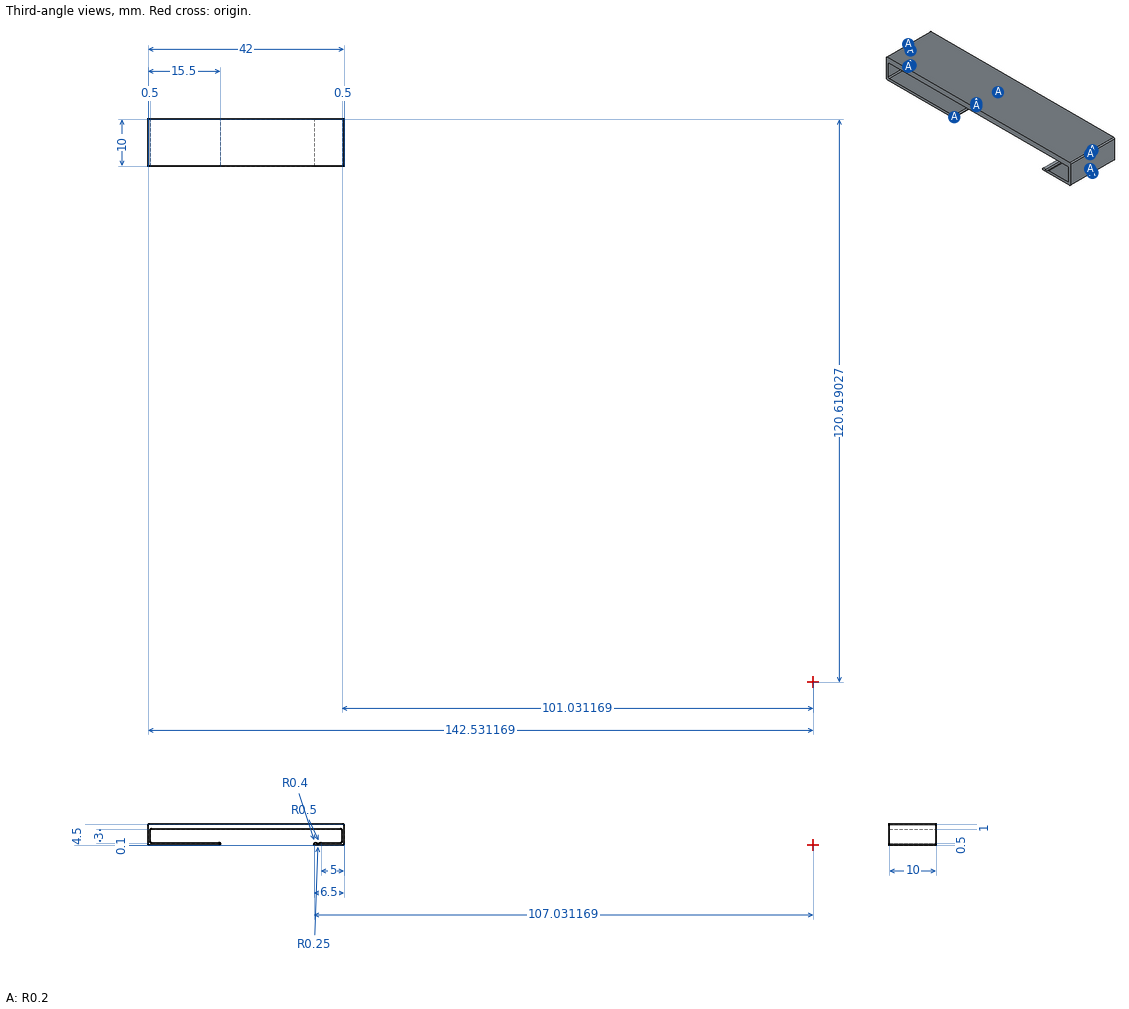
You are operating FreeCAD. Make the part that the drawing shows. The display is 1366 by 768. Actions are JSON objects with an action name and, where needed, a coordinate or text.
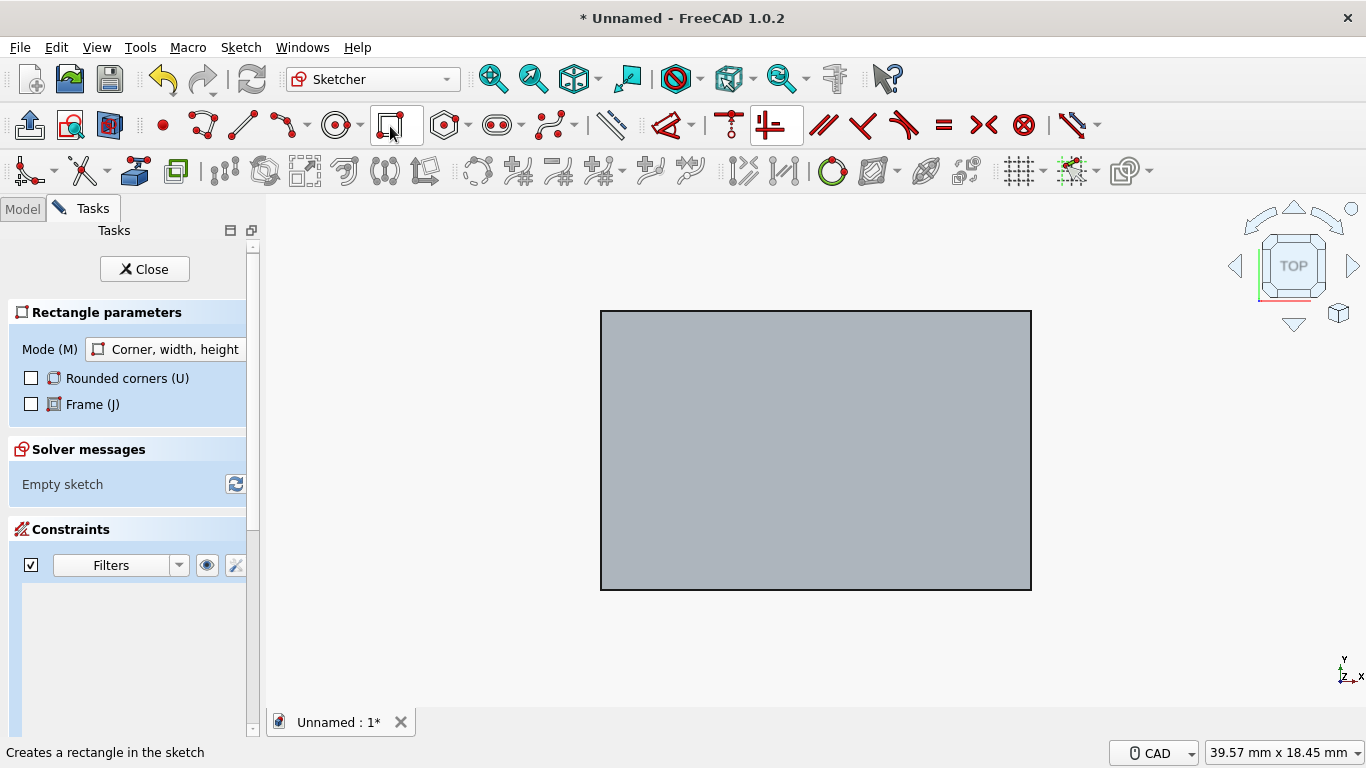
{"action": "left_click", "coordinate": [601, 311]}
{"action": "left_click", "coordinate": [614, 590]}
{"action": "key", "text": "Escape"}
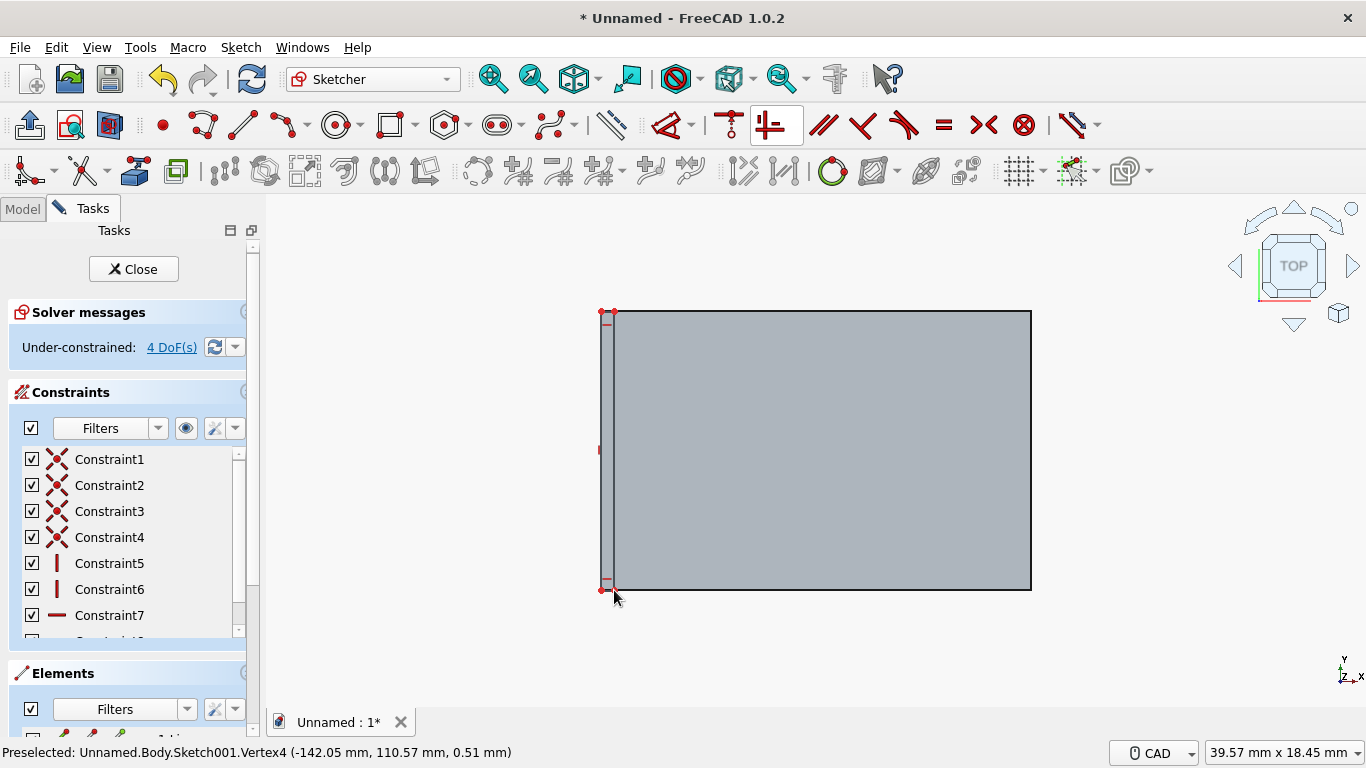
{"action": "left_click", "coordinate": [666, 126]}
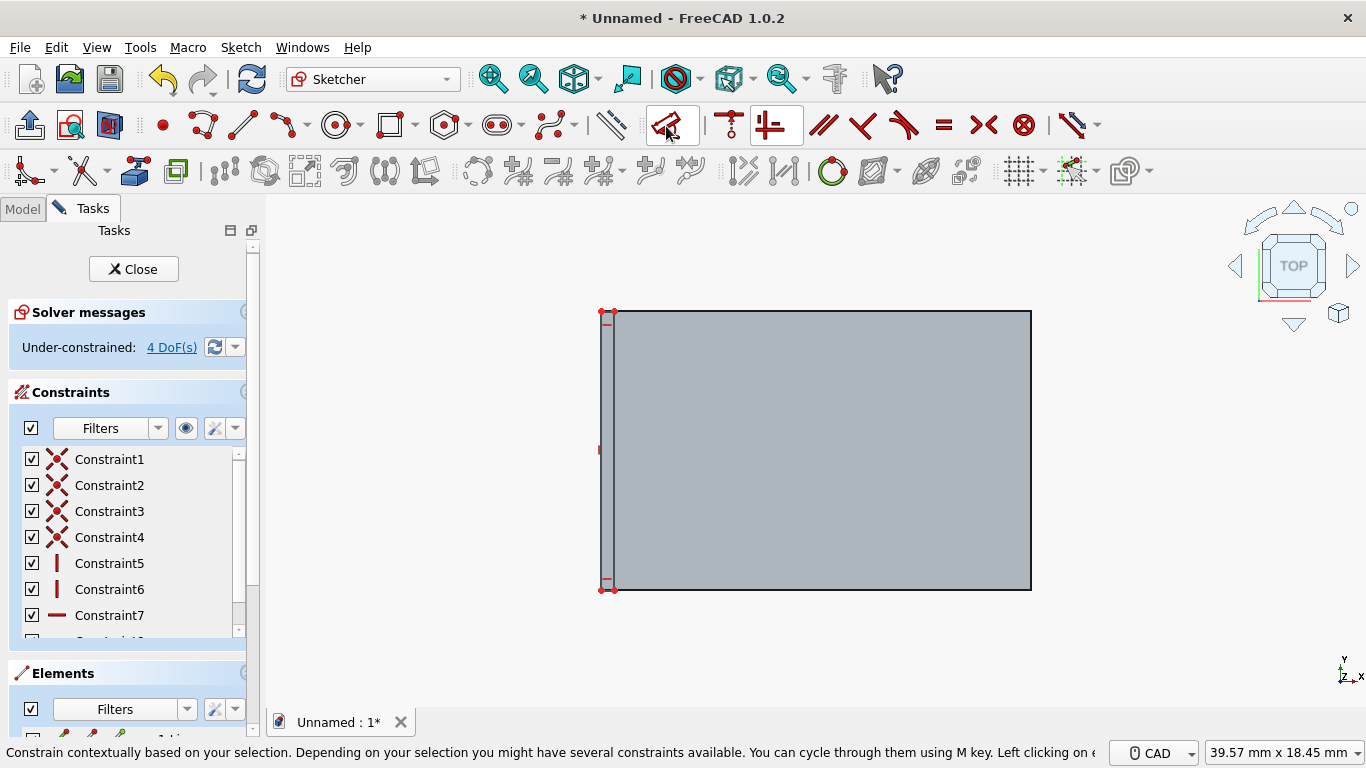
{"action": "left_click", "coordinate": [601, 396]}
{"action": "left_click", "coordinate": [567, 451]}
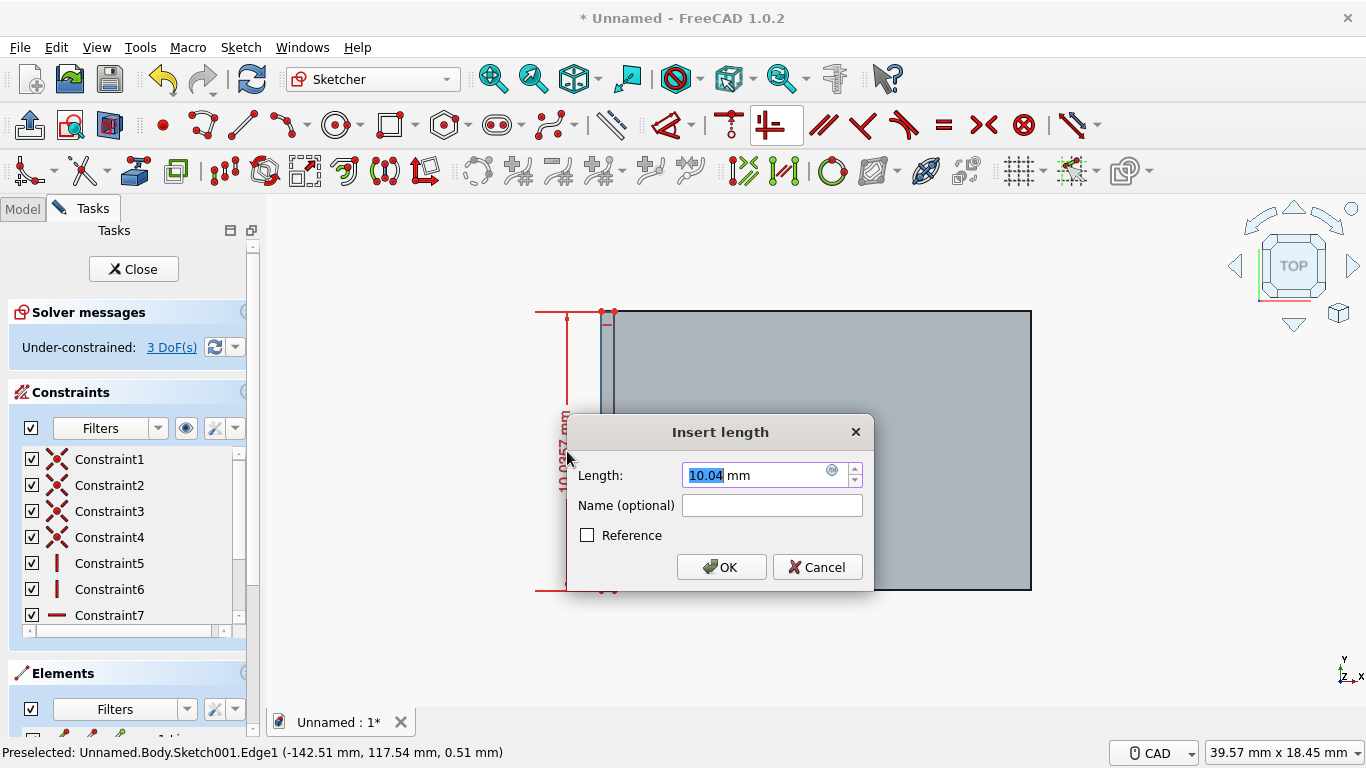
{"action": "type", "text": "10"}
{"action": "key", "text": "Return"}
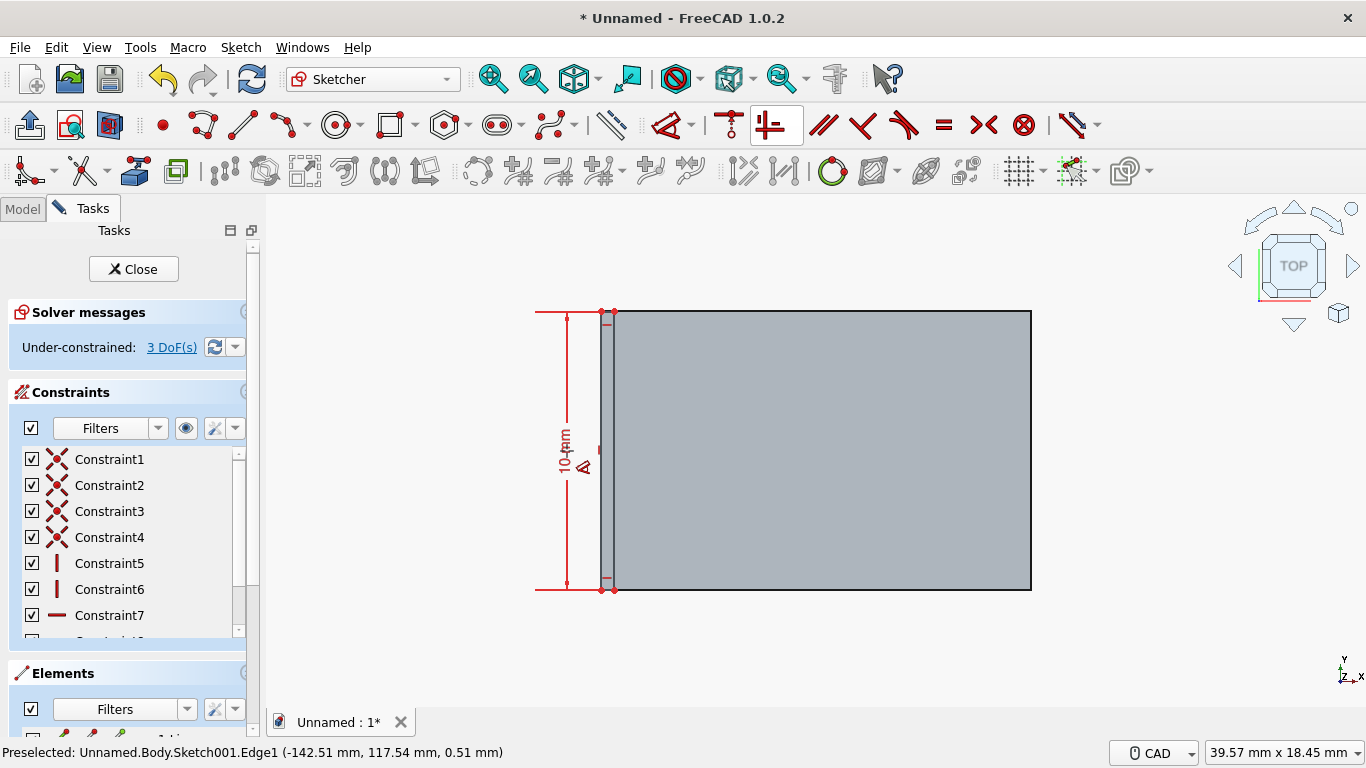
{"action": "scroll", "coordinate": [607, 590], "scroll_direction": "up", "scroll_amount": 6}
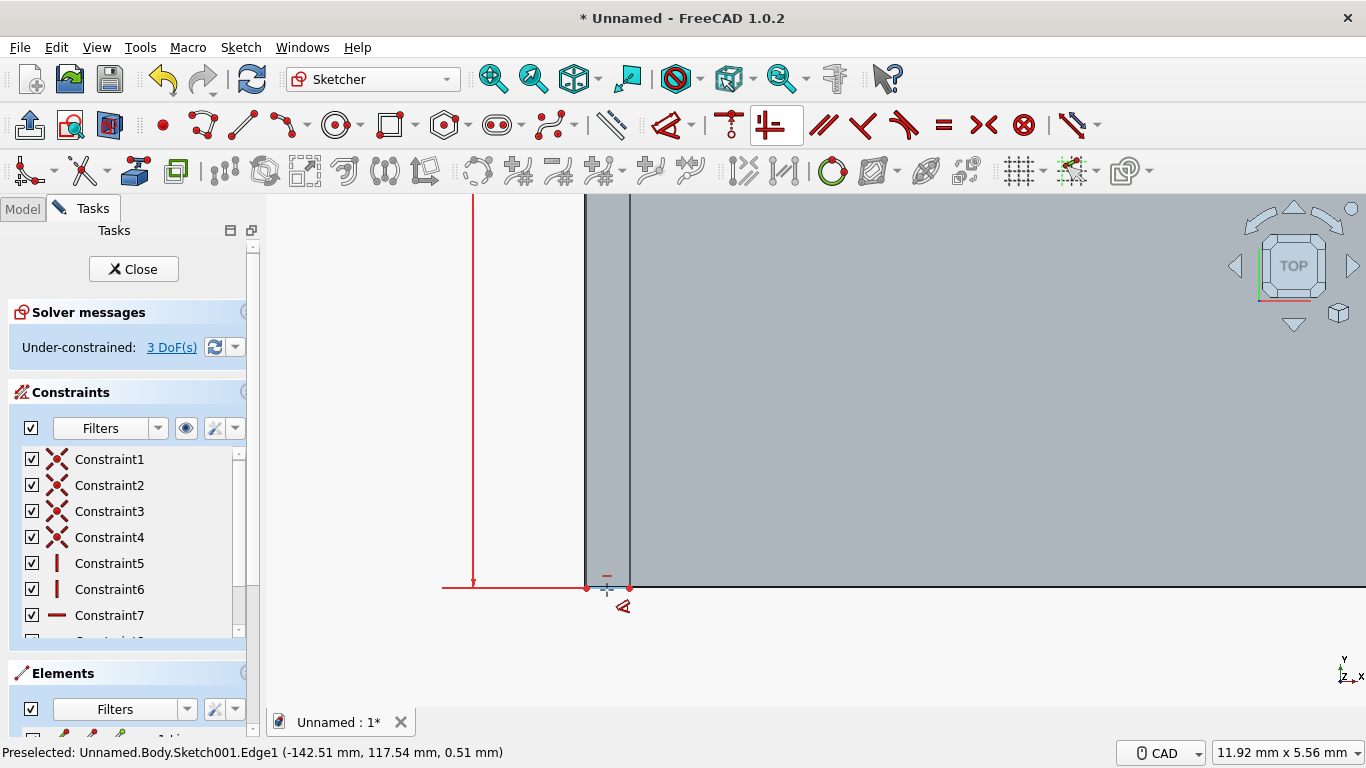
{"action": "left_click", "coordinate": [608, 588]}
{"action": "left_click", "coordinate": [608, 622]}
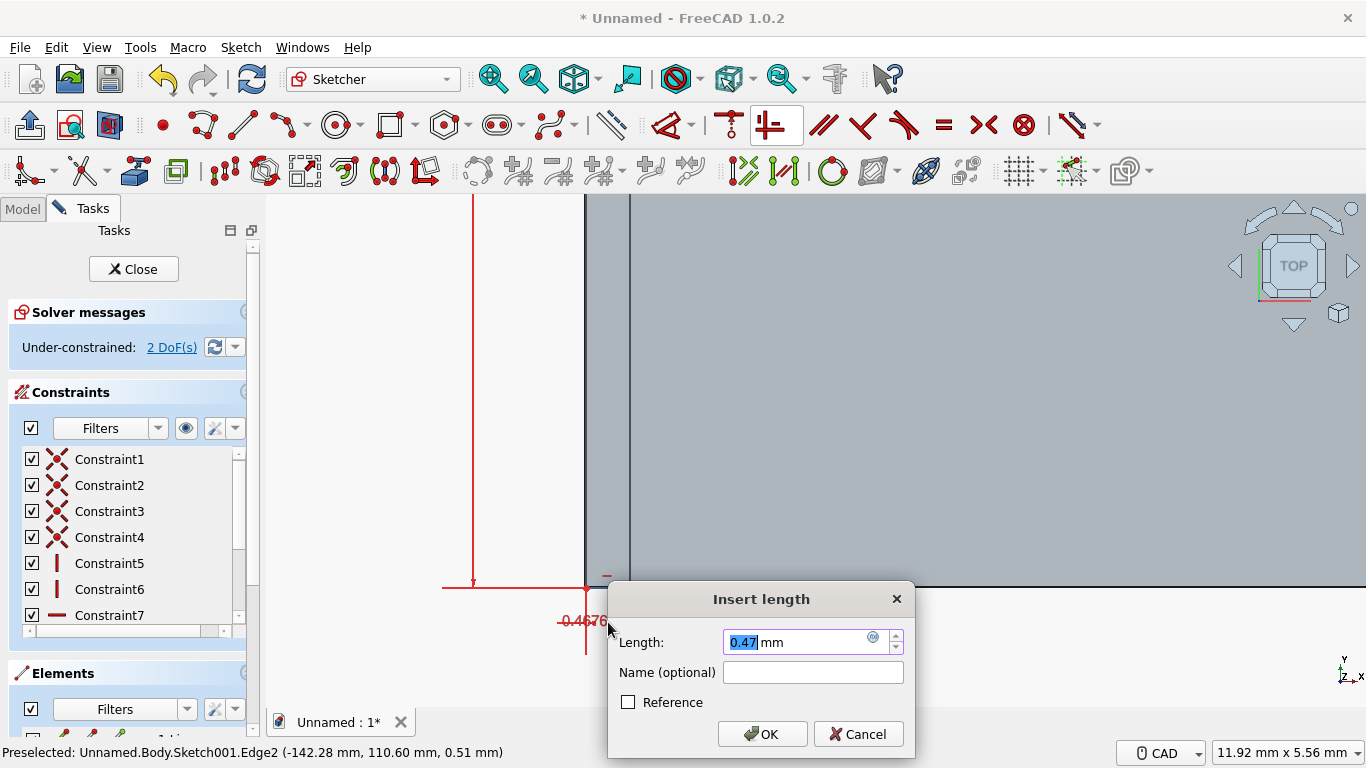
{"action": "type", "text": "0.5"}
{"action": "key", "text": "Return"}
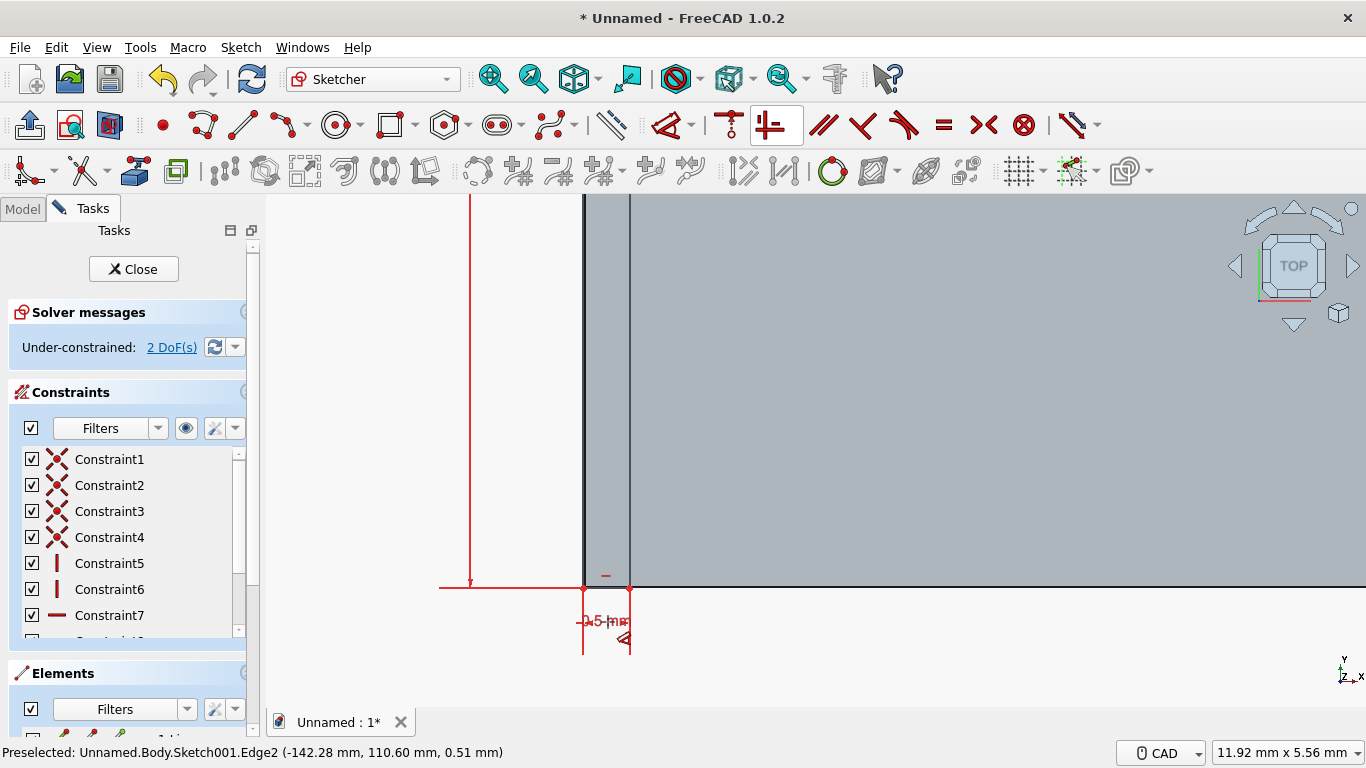
{"action": "scroll", "coordinate": [829, 640], "scroll_direction": "down", "scroll_amount": 5}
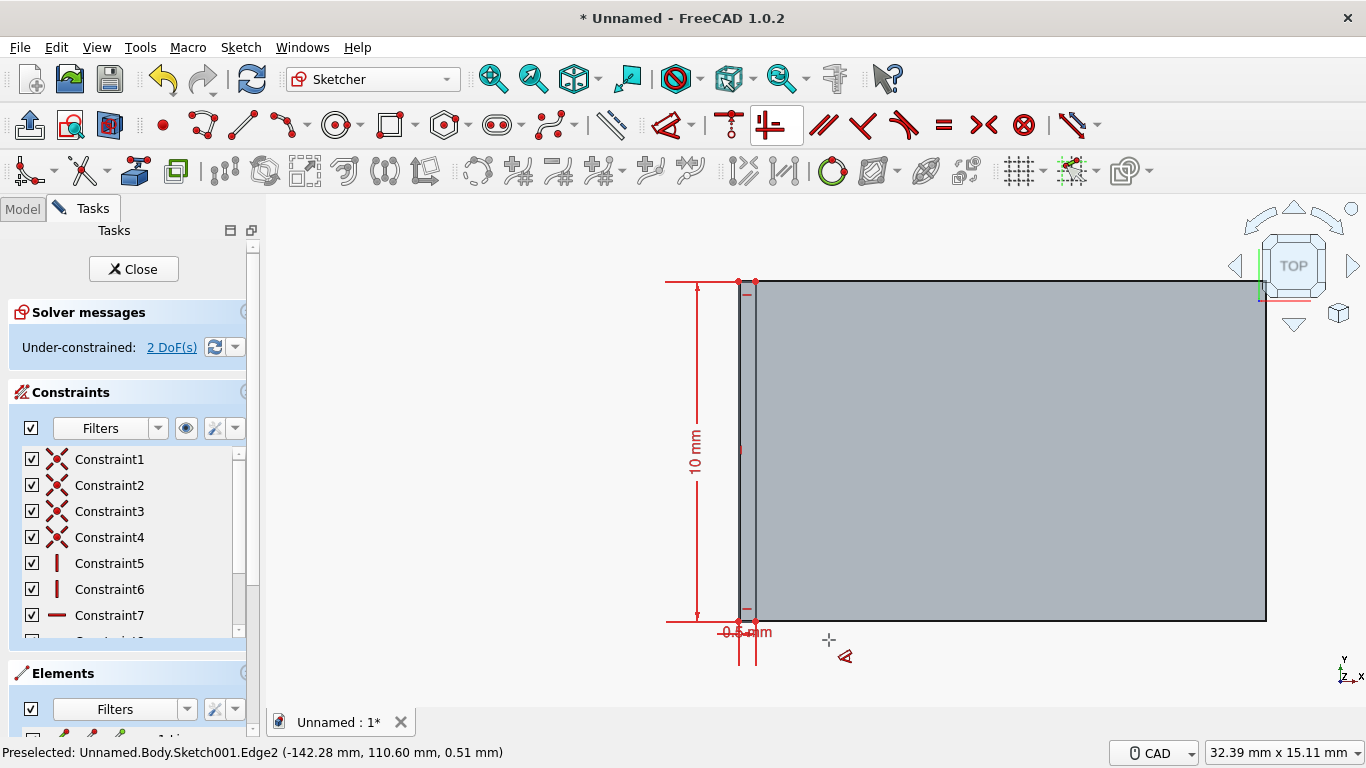
{"action": "left_click", "coordinate": [739, 282]}
{"action": "left_click", "coordinate": [970, 248]}